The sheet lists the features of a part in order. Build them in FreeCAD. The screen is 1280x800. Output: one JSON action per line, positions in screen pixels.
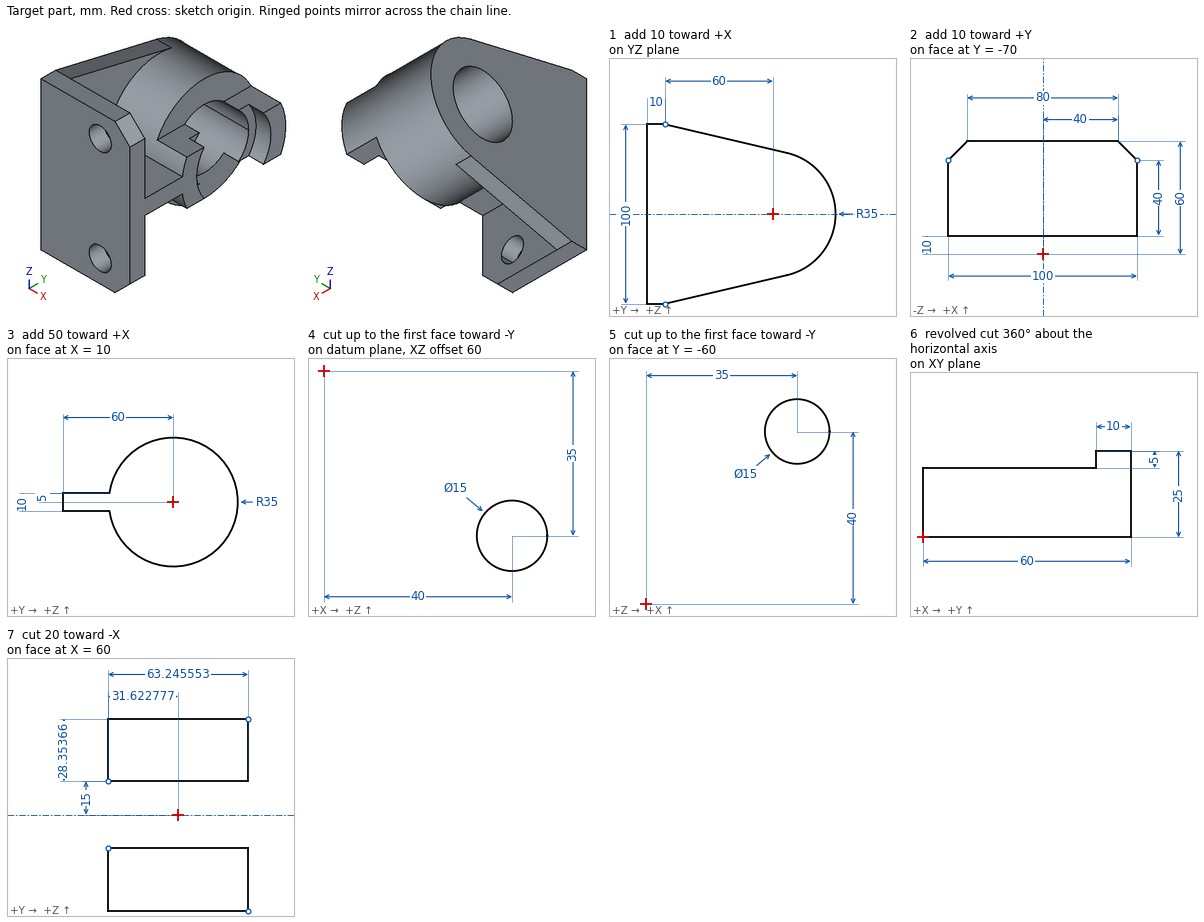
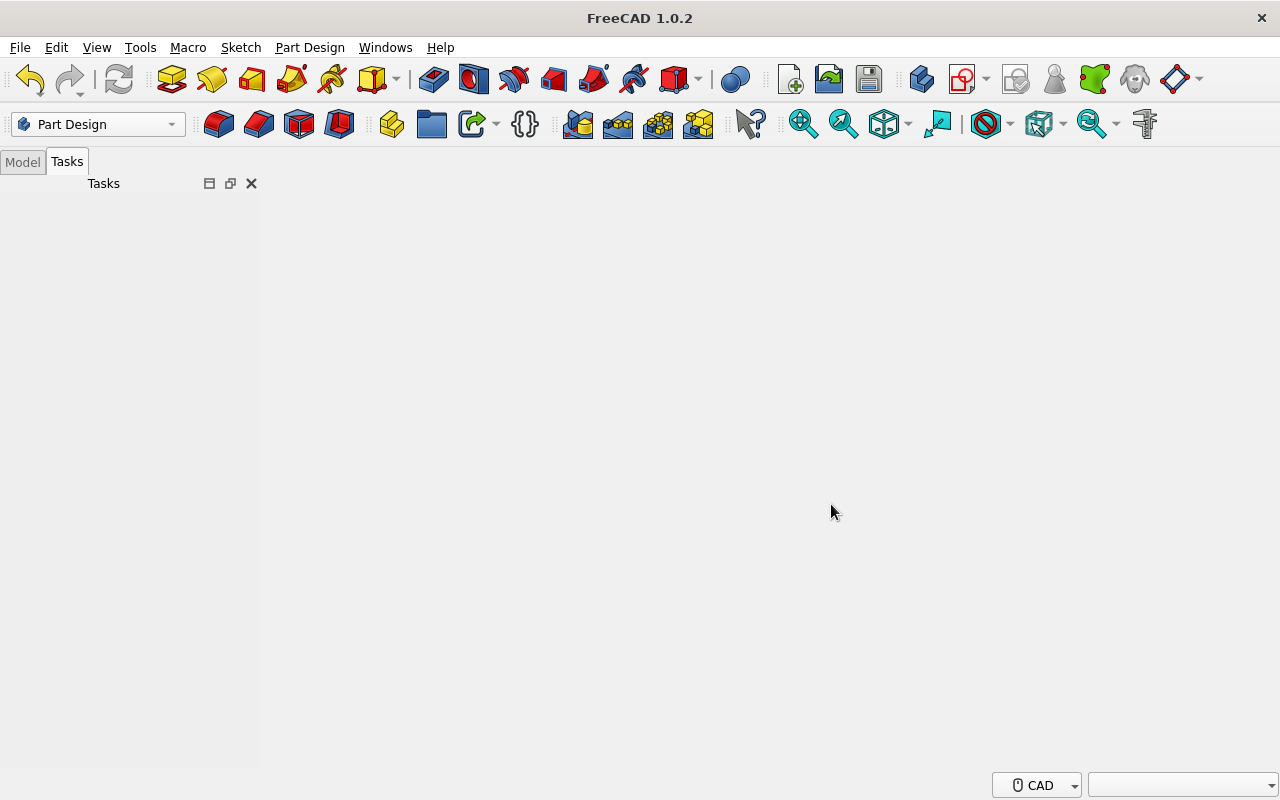
{"action": "left_click", "coordinate": [790, 80]}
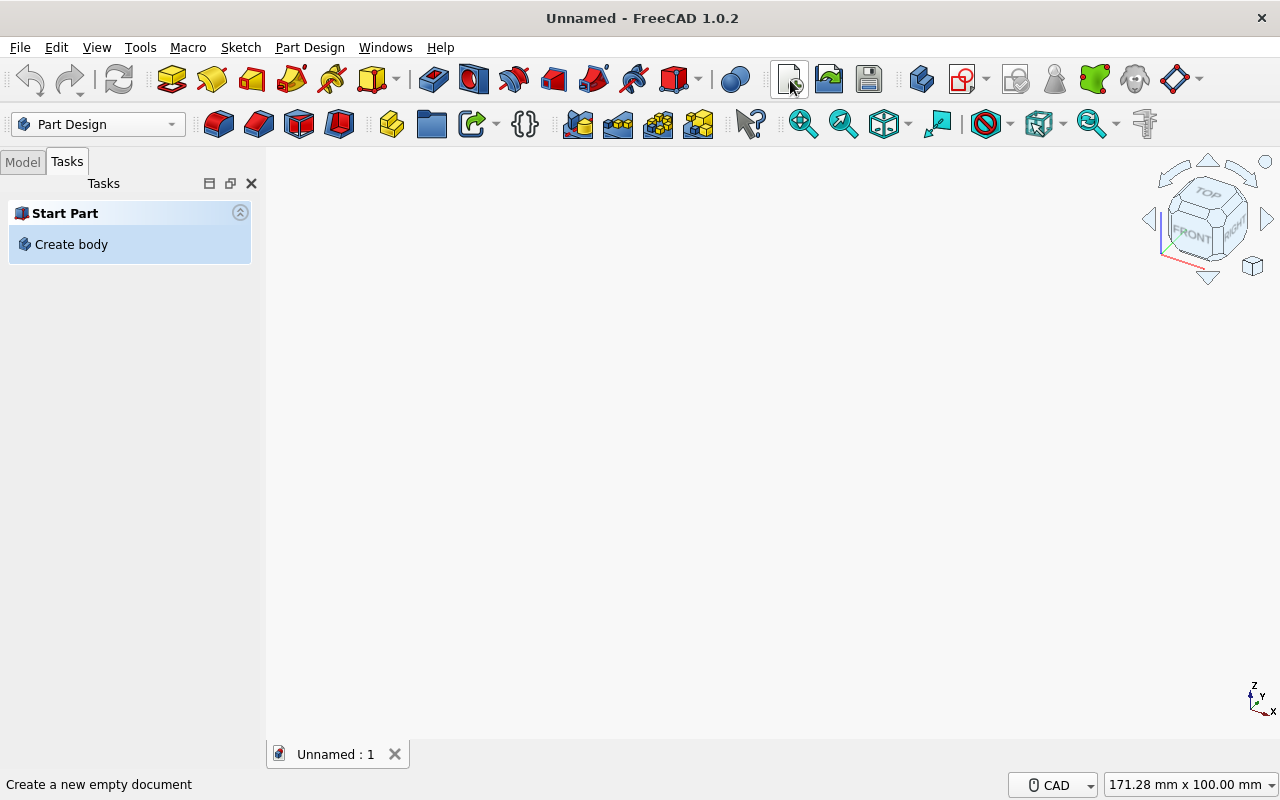
{"action": "left_click", "coordinate": [962, 80]}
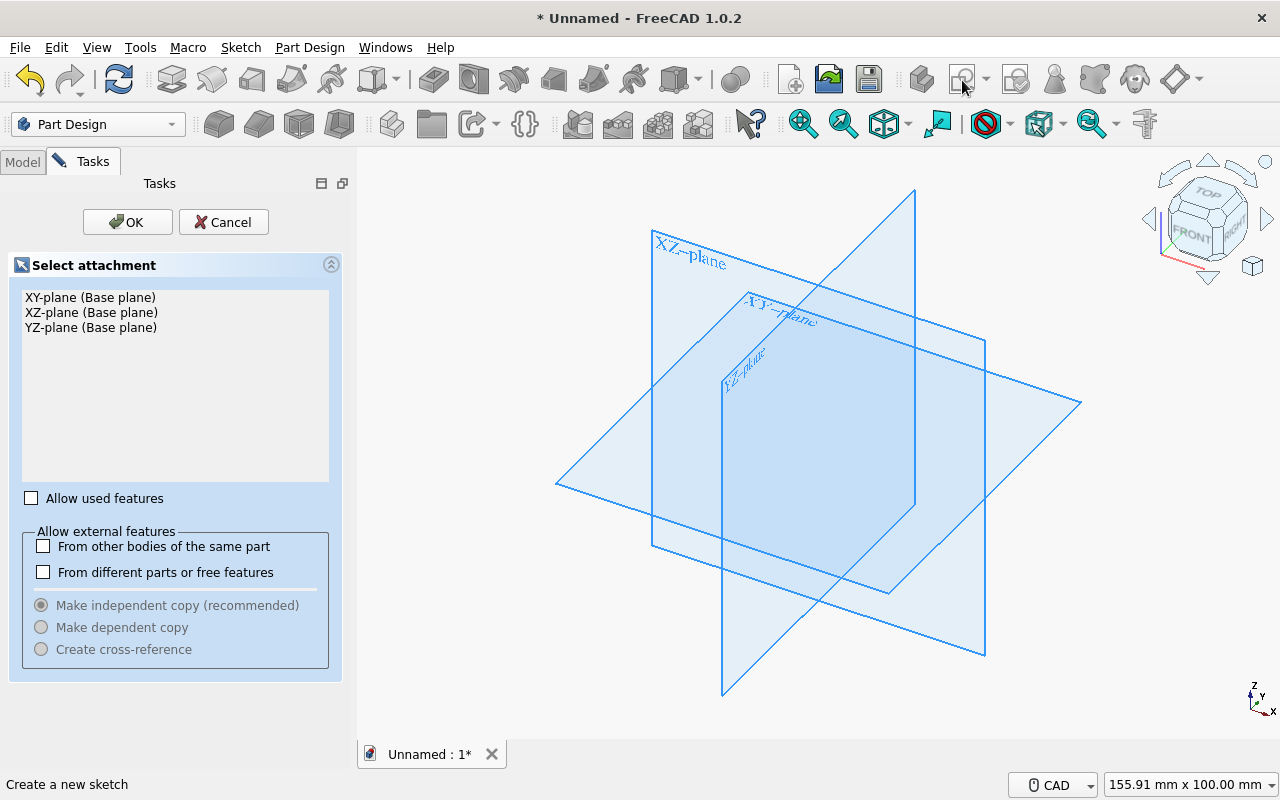
{"action": "left_click", "coordinate": [82, 328]}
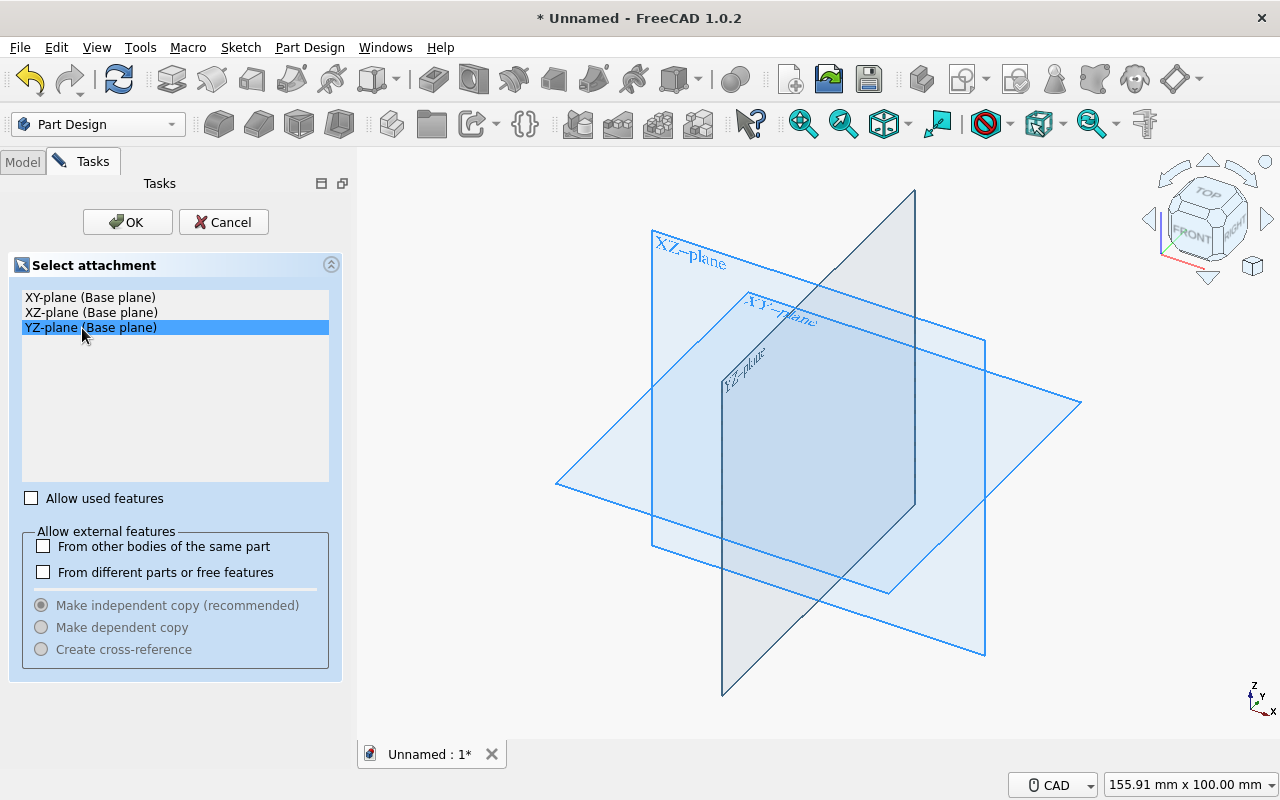
{"action": "left_click", "coordinate": [128, 222]}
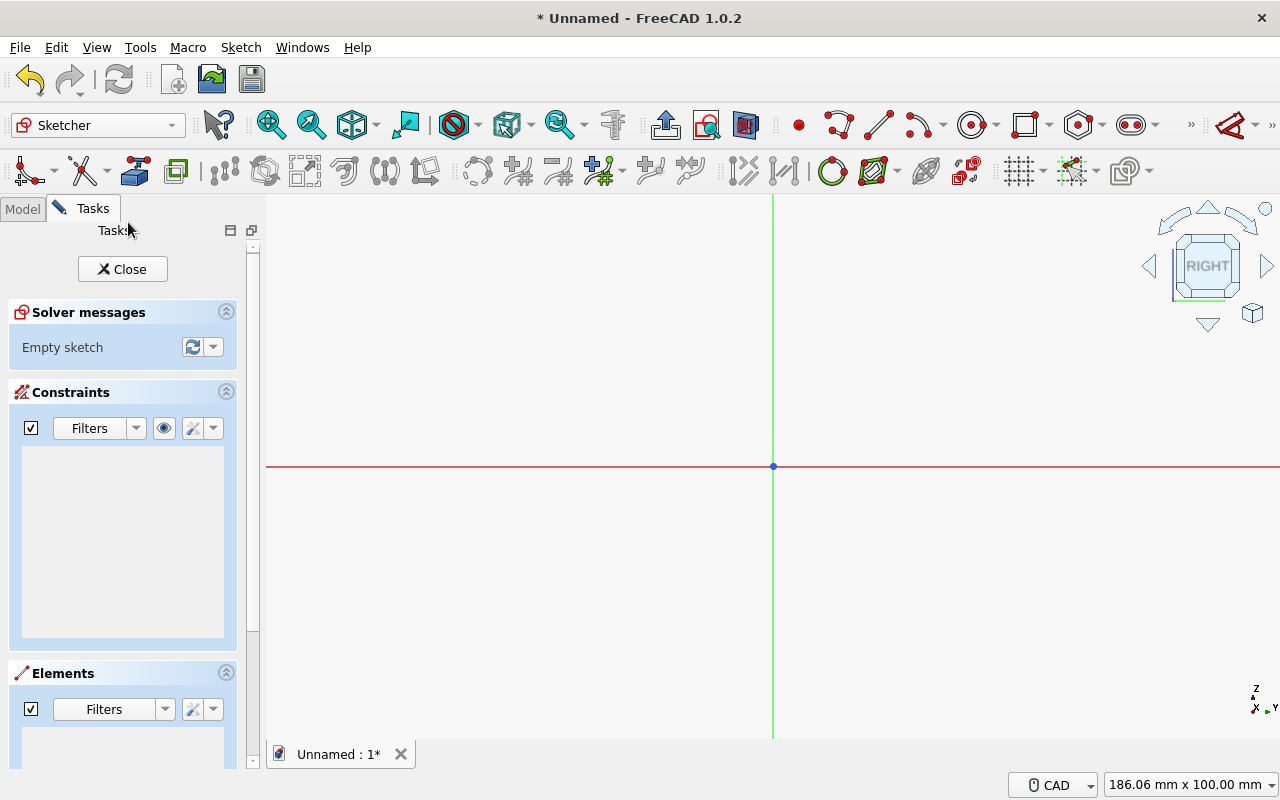
{"action": "scroll", "coordinate": [759, 466], "scroll_direction": "down", "scroll_amount": 2}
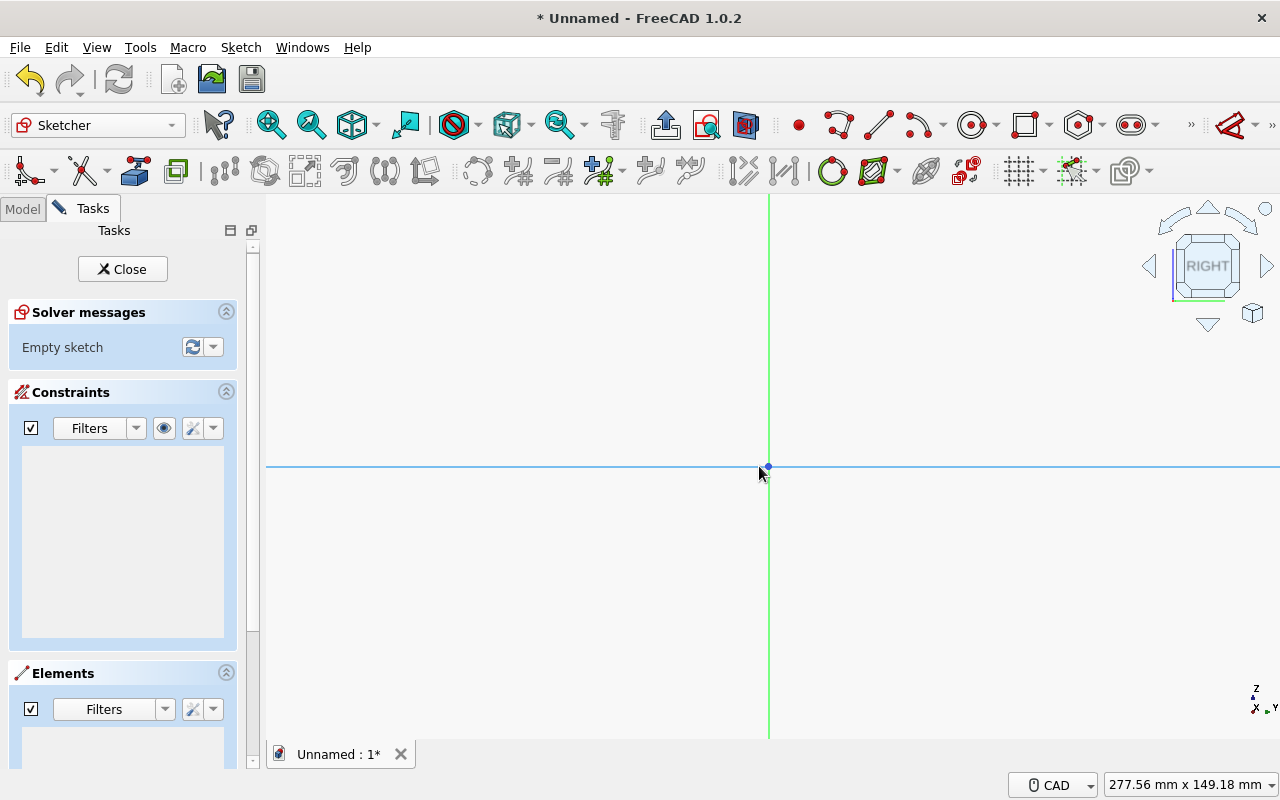
{"action": "left_click", "coordinate": [840, 126]}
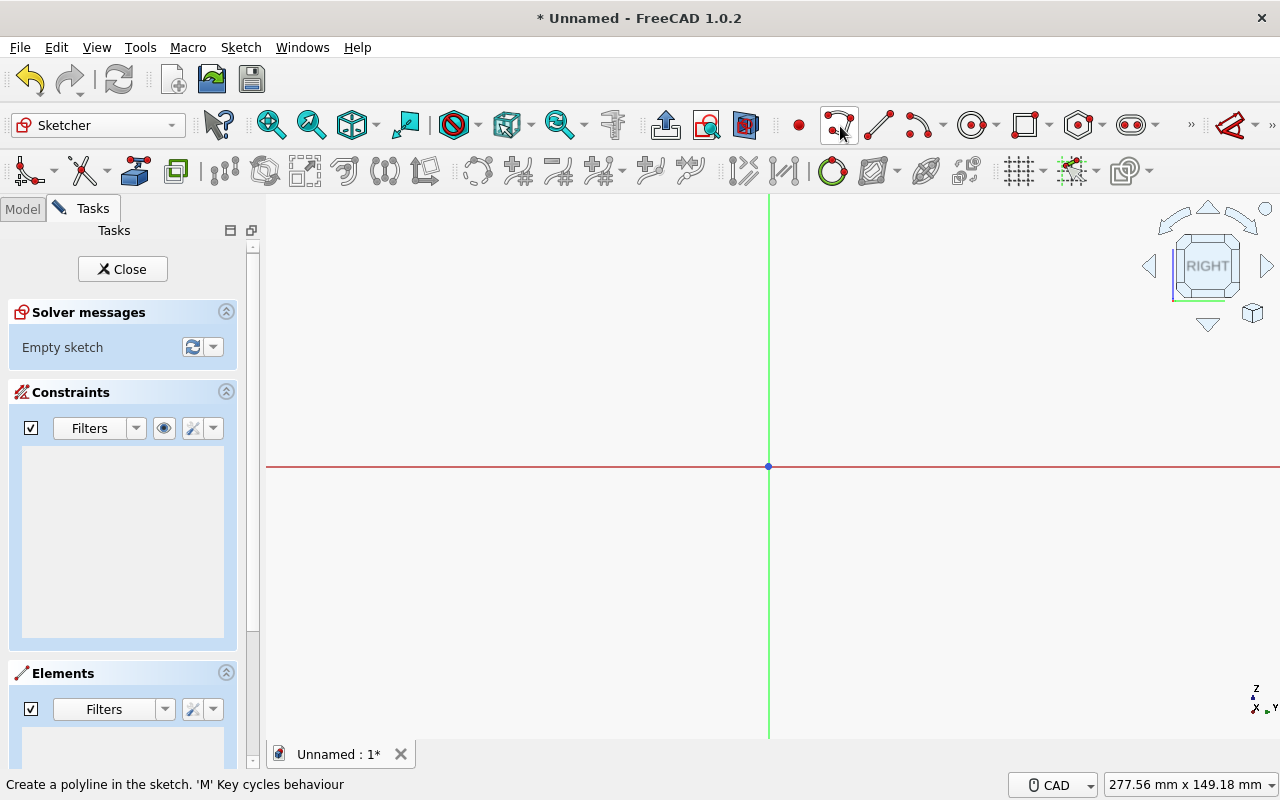
{"action": "left_click", "coordinate": [798, 342]}
{"action": "left_click", "coordinate": [549, 284]}
{"action": "left_click", "coordinate": [513, 284]}
{"action": "left_click", "coordinate": [513, 649]}
{"action": "left_click", "coordinate": [549, 649]}
{"action": "left_click", "coordinate": [798, 591]}
{"action": "right_click", "coordinate": [798, 591]}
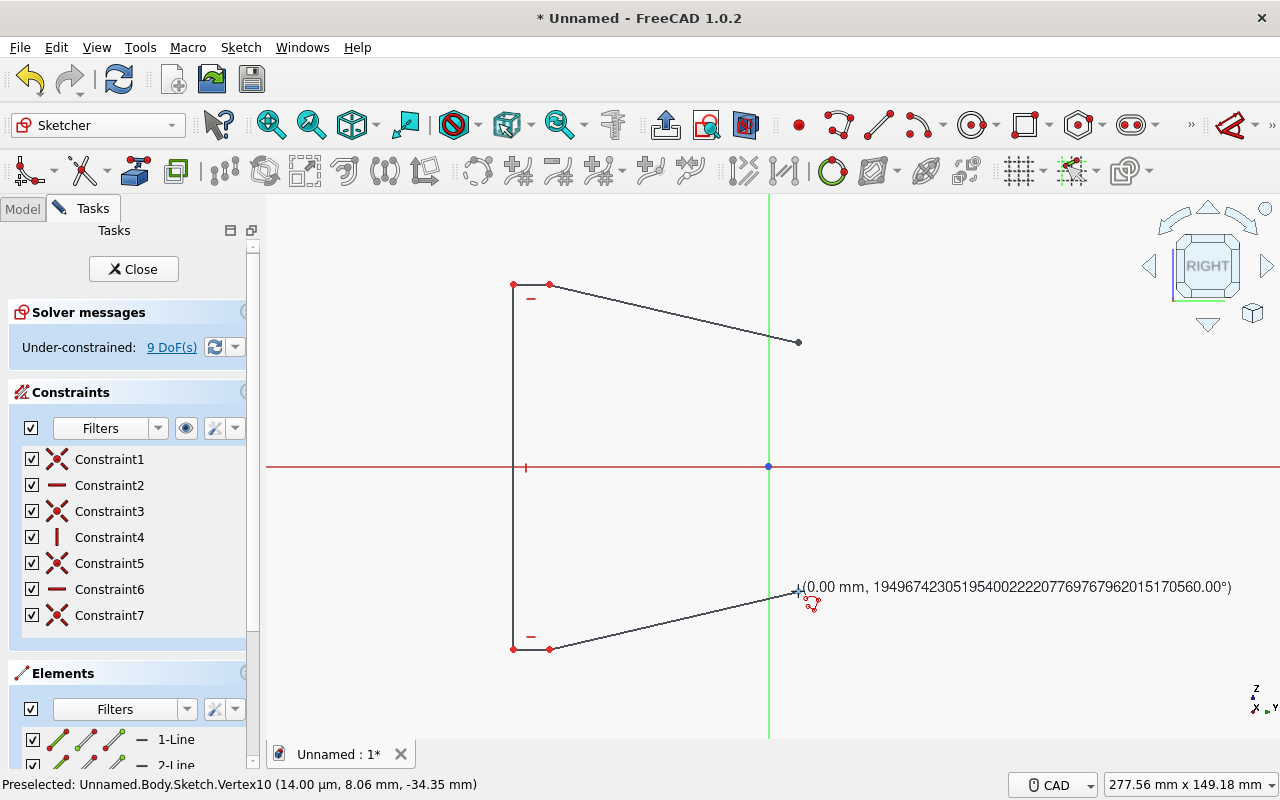
{"action": "left_click", "coordinate": [946, 126]}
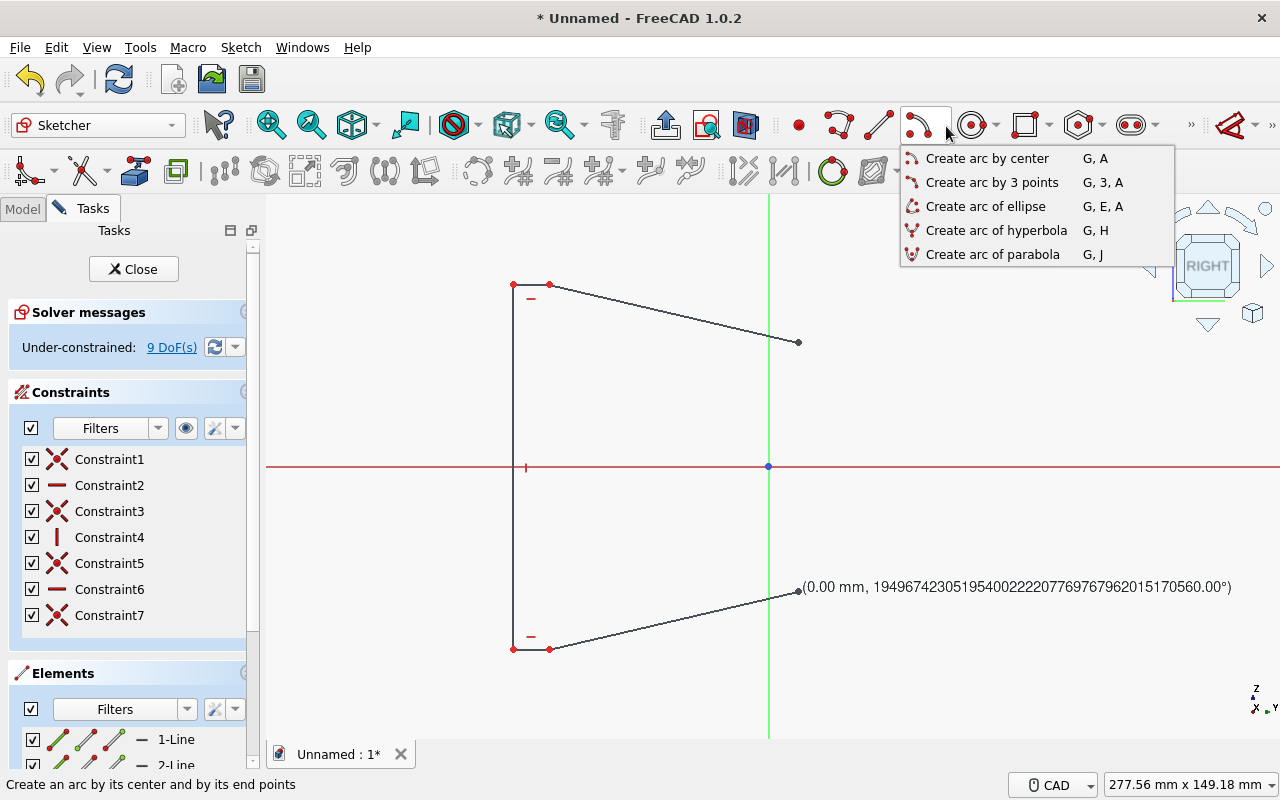
{"action": "left_click", "coordinate": [1038, 182]}